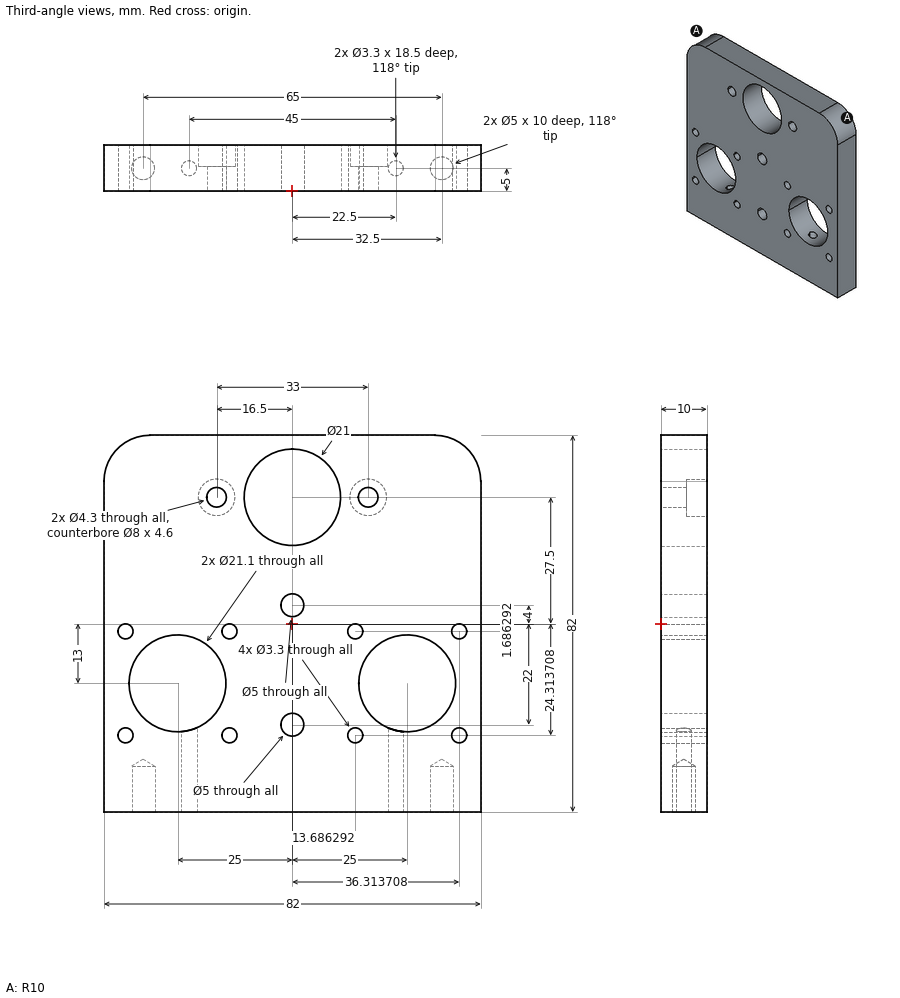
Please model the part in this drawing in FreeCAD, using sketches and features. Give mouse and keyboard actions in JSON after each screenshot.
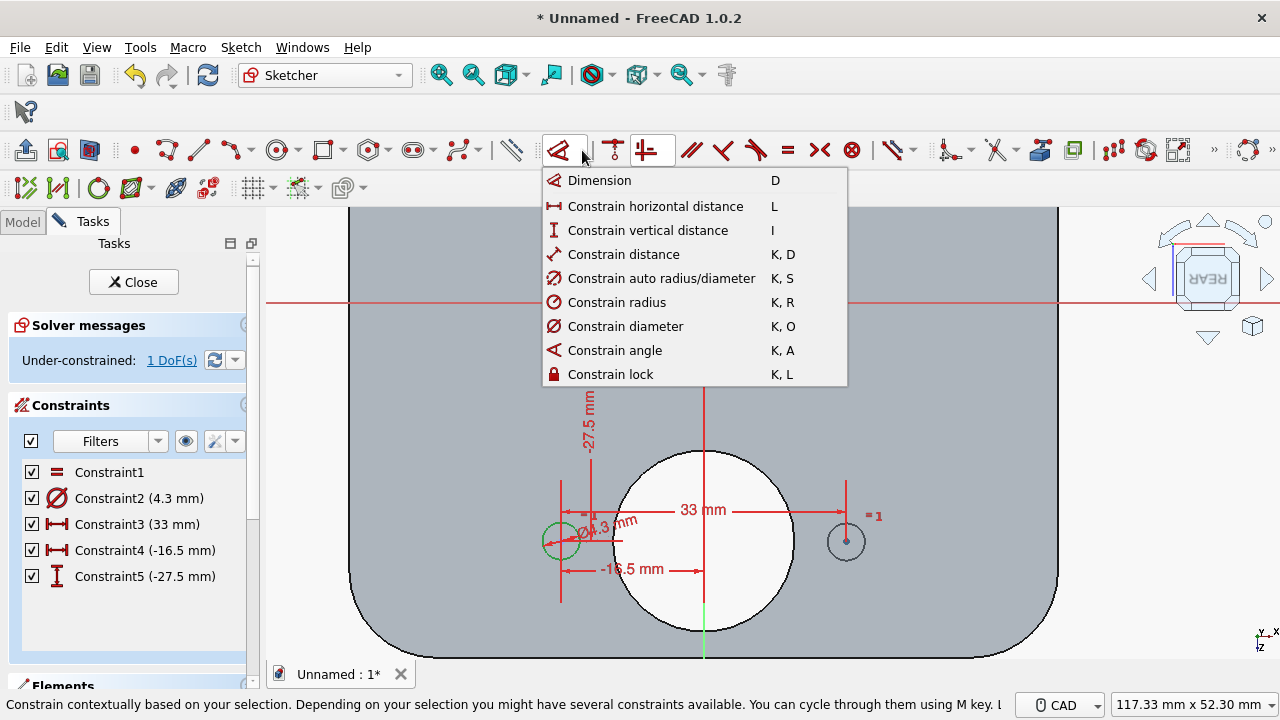
{"action": "left_click", "coordinate": [695, 230]}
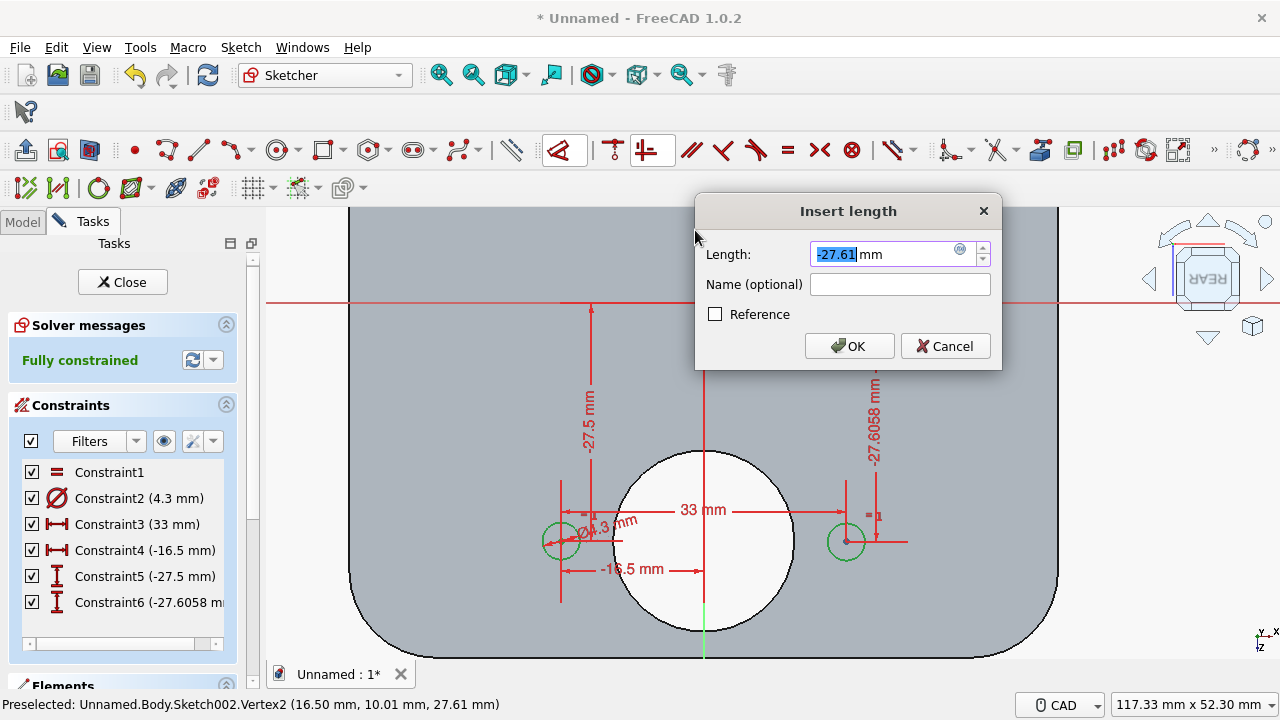
{"action": "type", "text": "-27.5"}
{"action": "key", "text": "Return"}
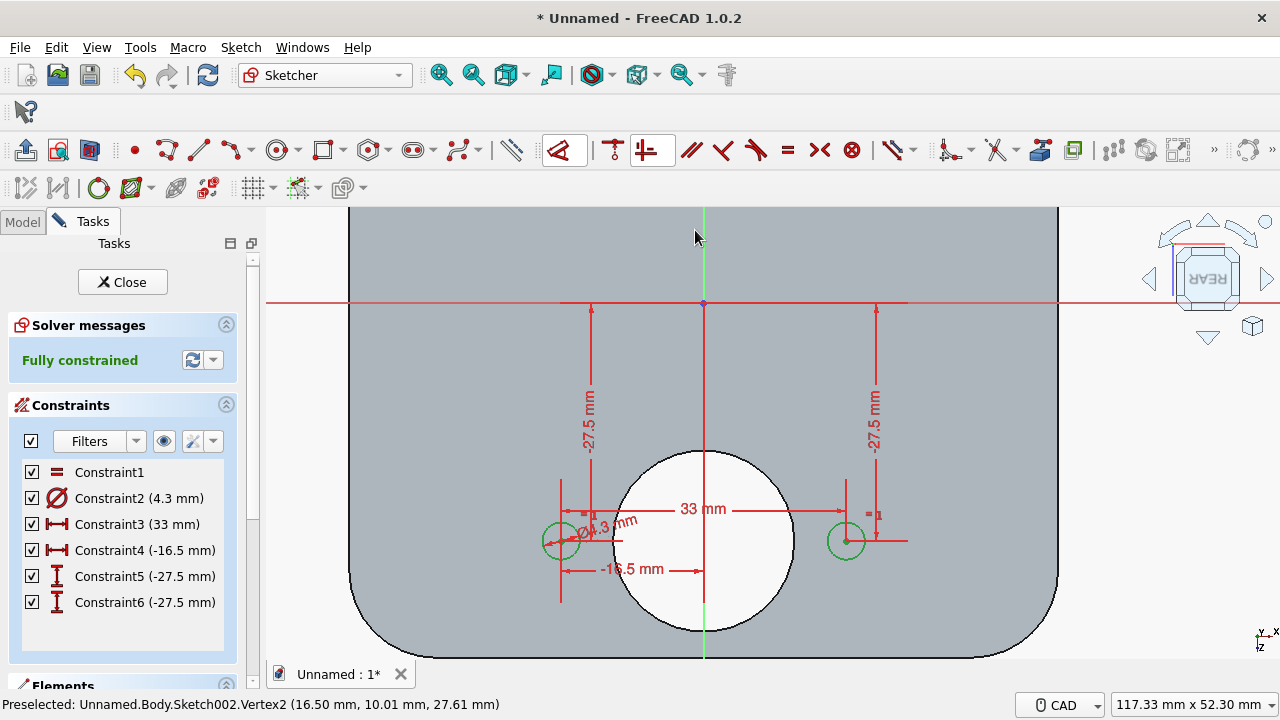
{"action": "left_click", "coordinate": [123, 282]}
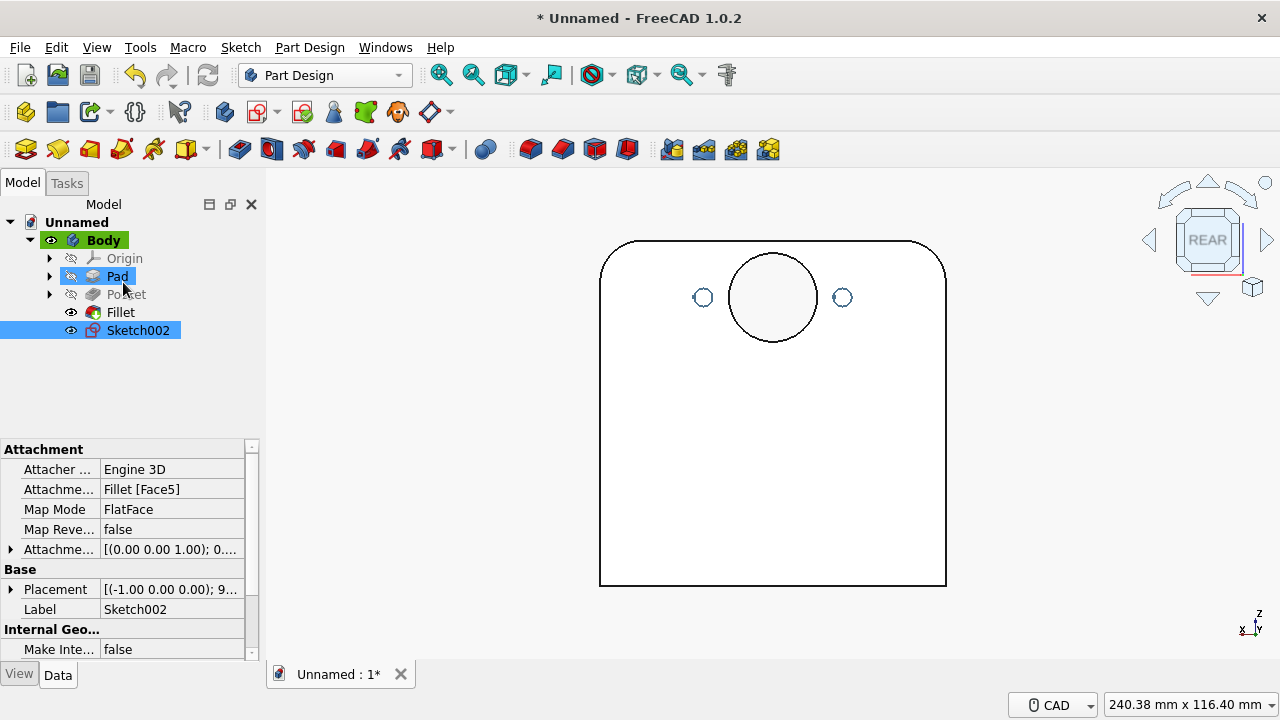
{"action": "left_click", "coordinate": [272, 150]}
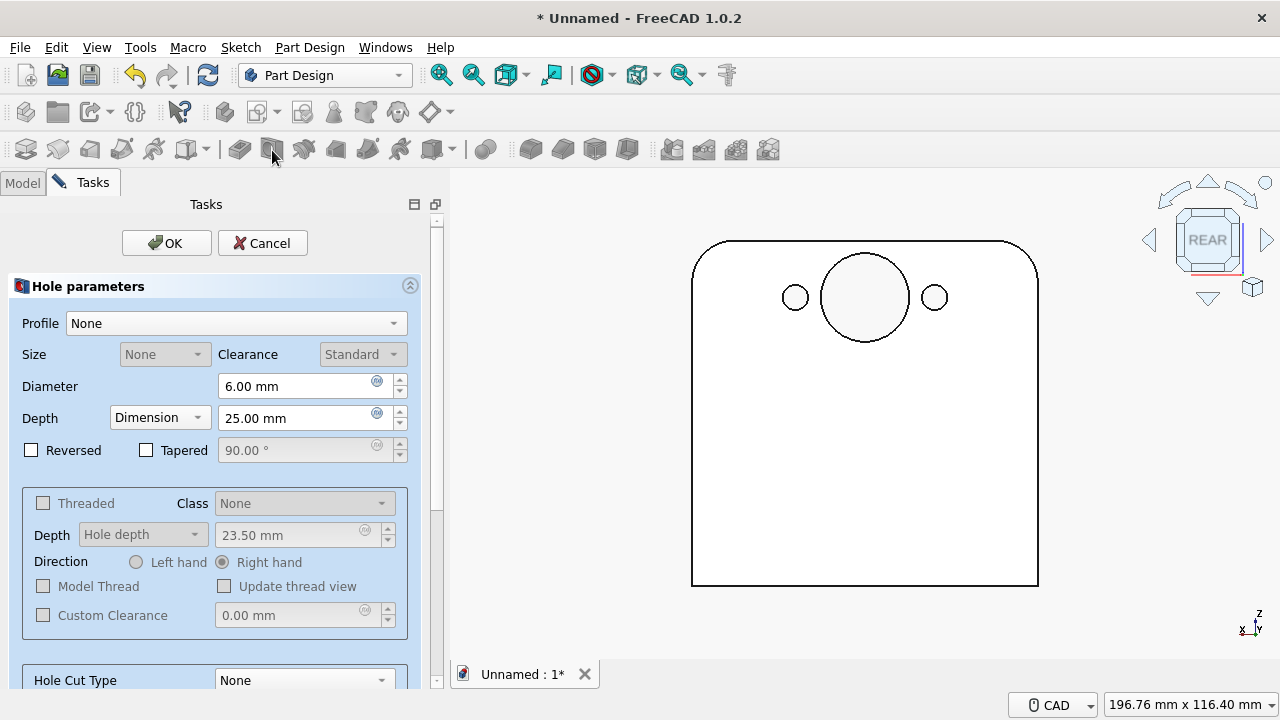
{"action": "triple_click", "coordinate": [305, 386]}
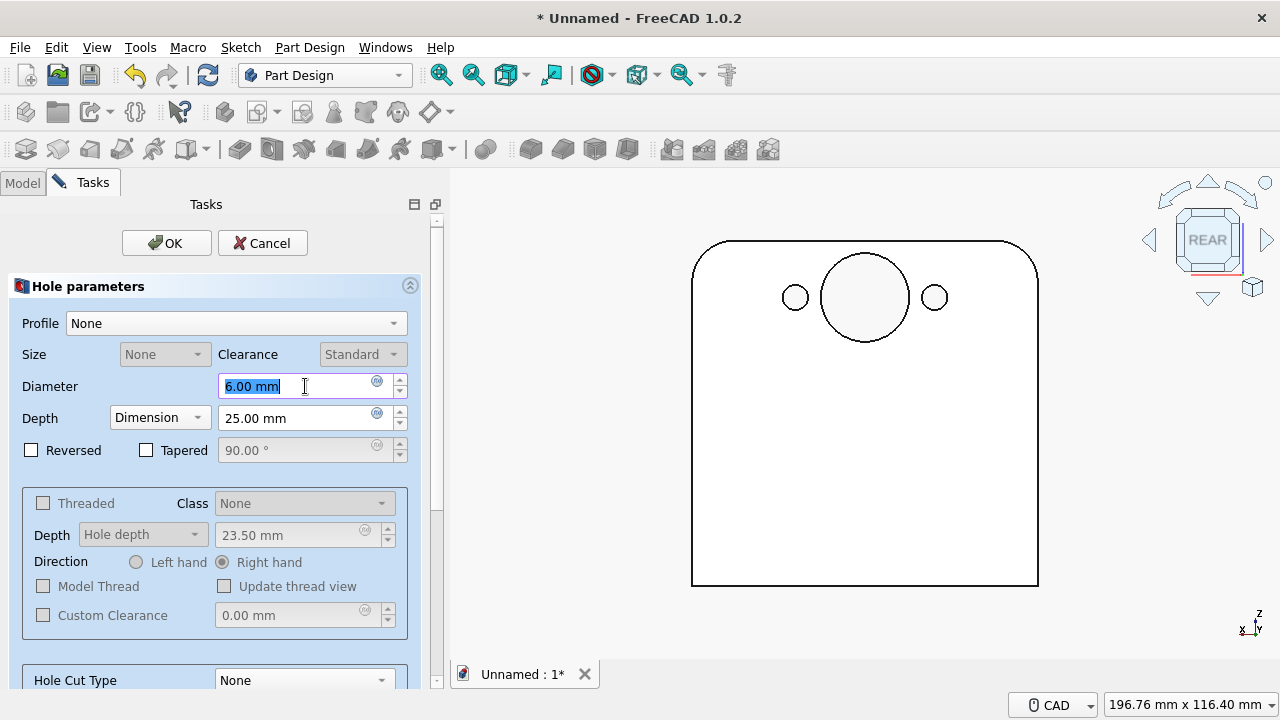
{"action": "type", "text": "4.3"}
{"action": "key", "text": "Tab"}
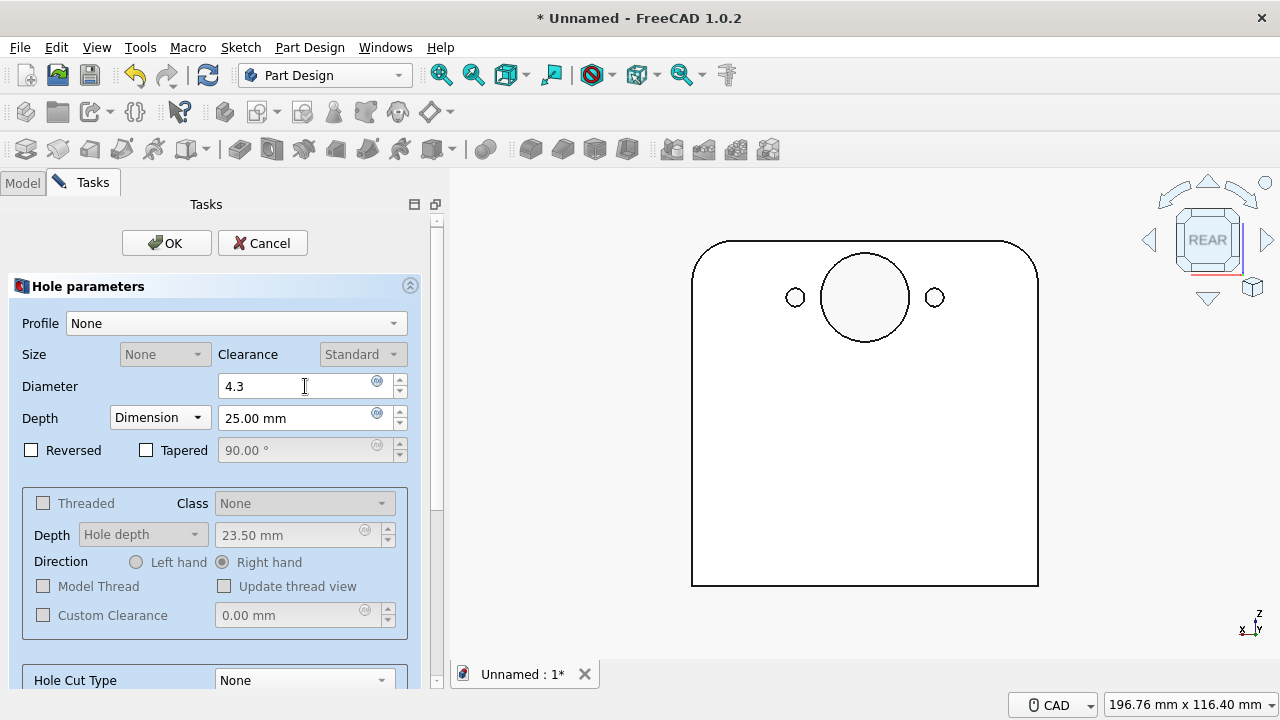
{"action": "left_click", "coordinate": [161, 418]}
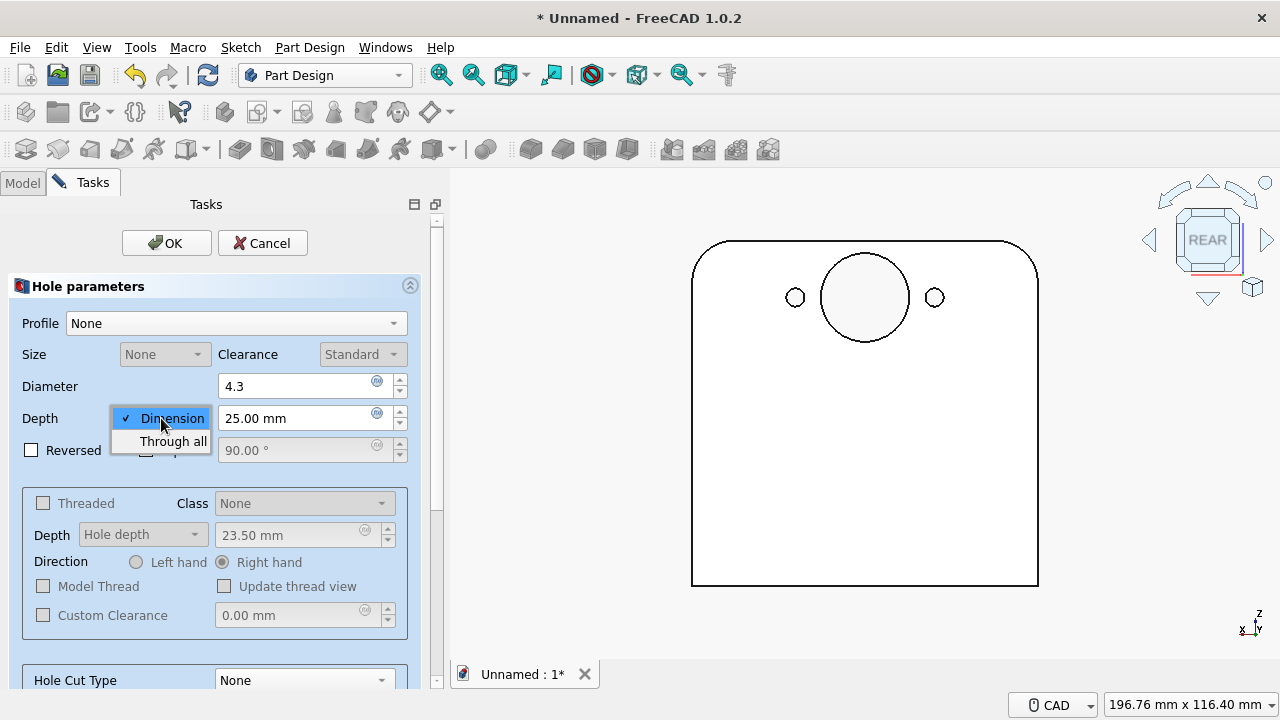
{"action": "left_click", "coordinate": [160, 442]}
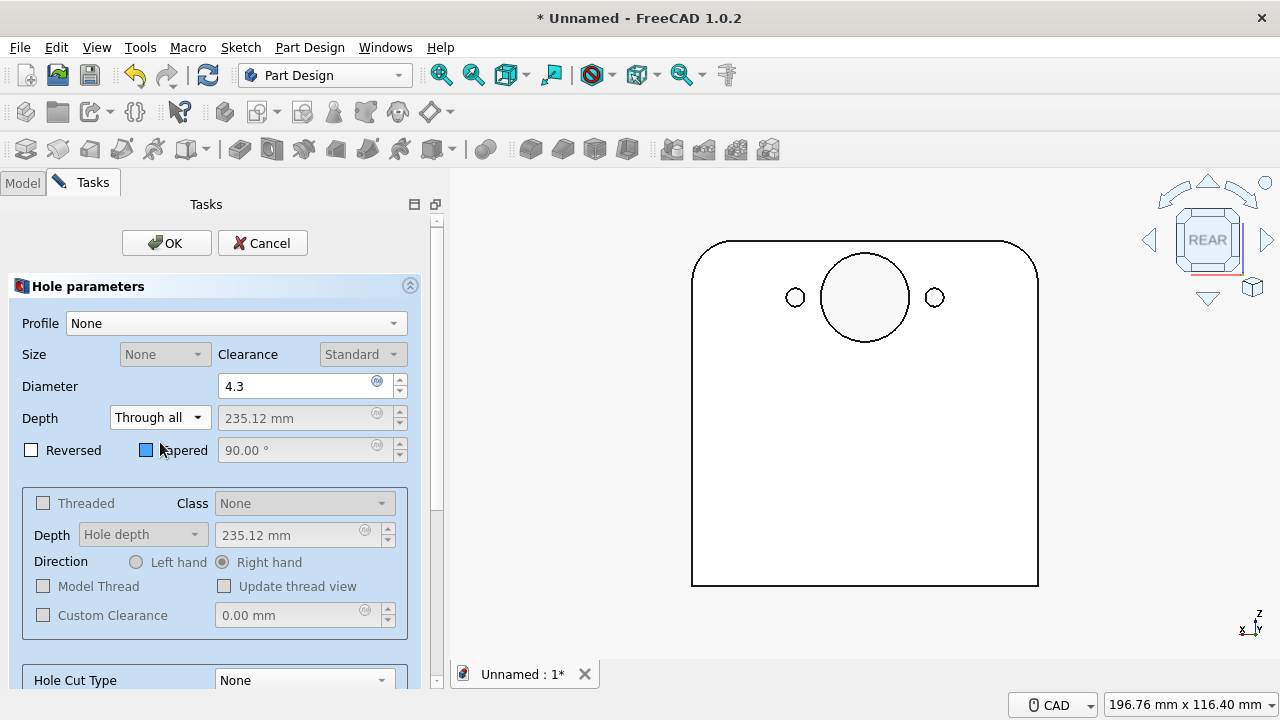
{"action": "scroll", "coordinate": [437, 451], "scroll_direction": "down", "scroll_amount": 2}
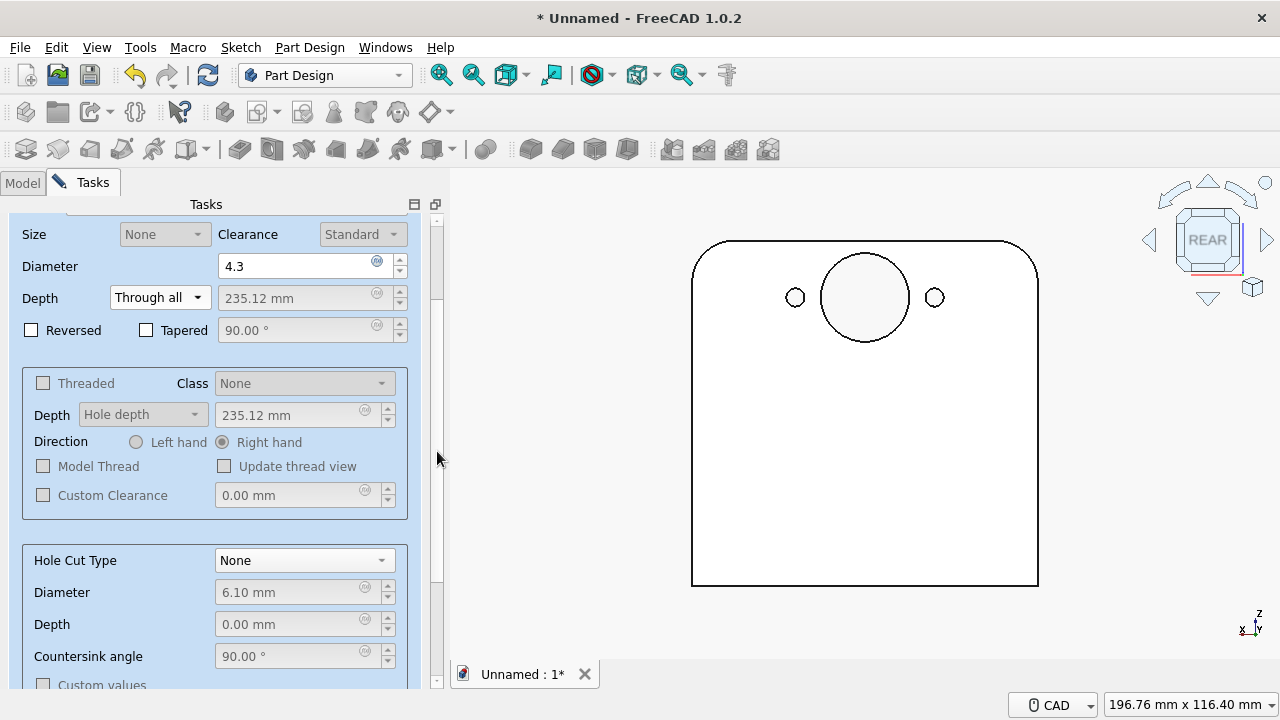
{"action": "left_click", "coordinate": [306, 560]}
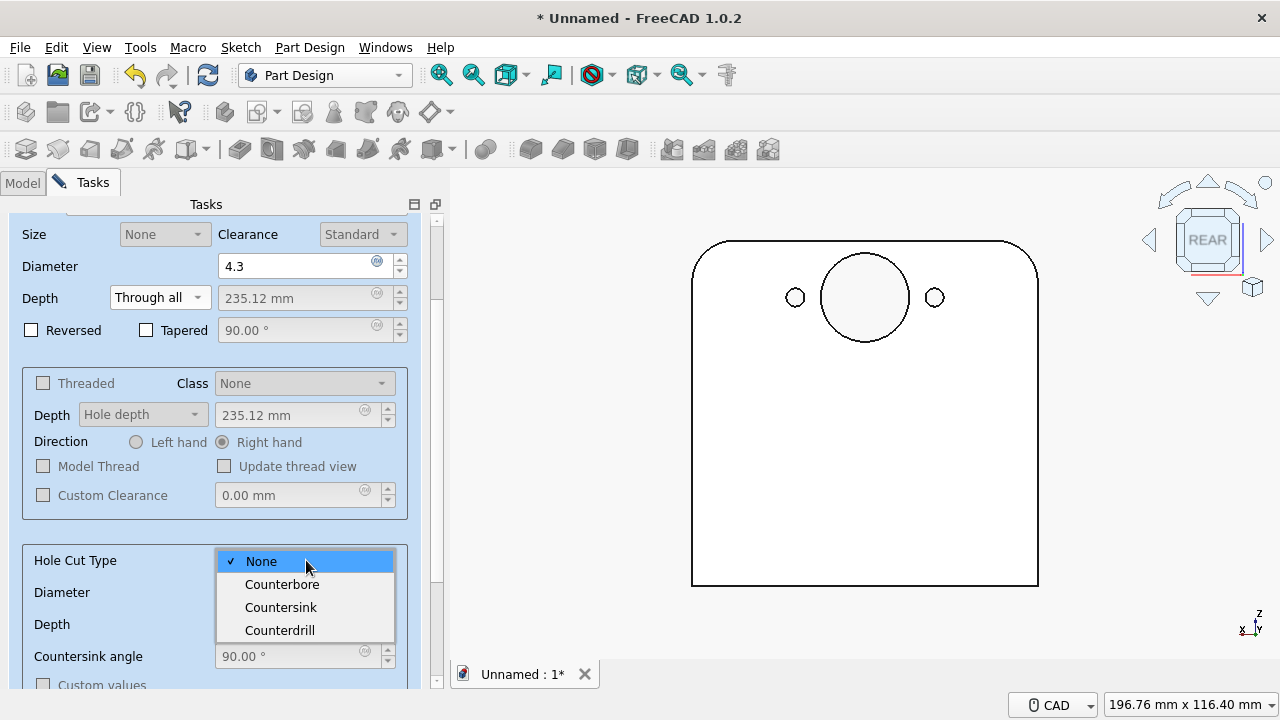
{"action": "left_click", "coordinate": [304, 584]}